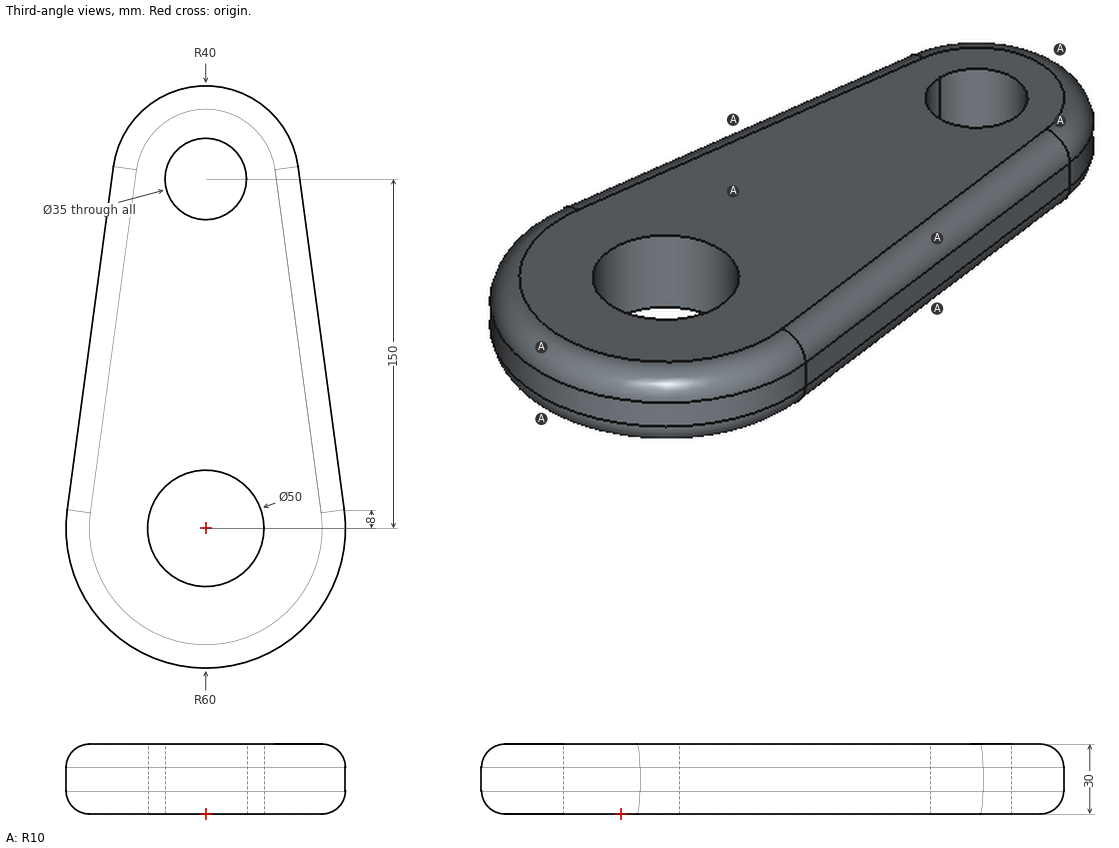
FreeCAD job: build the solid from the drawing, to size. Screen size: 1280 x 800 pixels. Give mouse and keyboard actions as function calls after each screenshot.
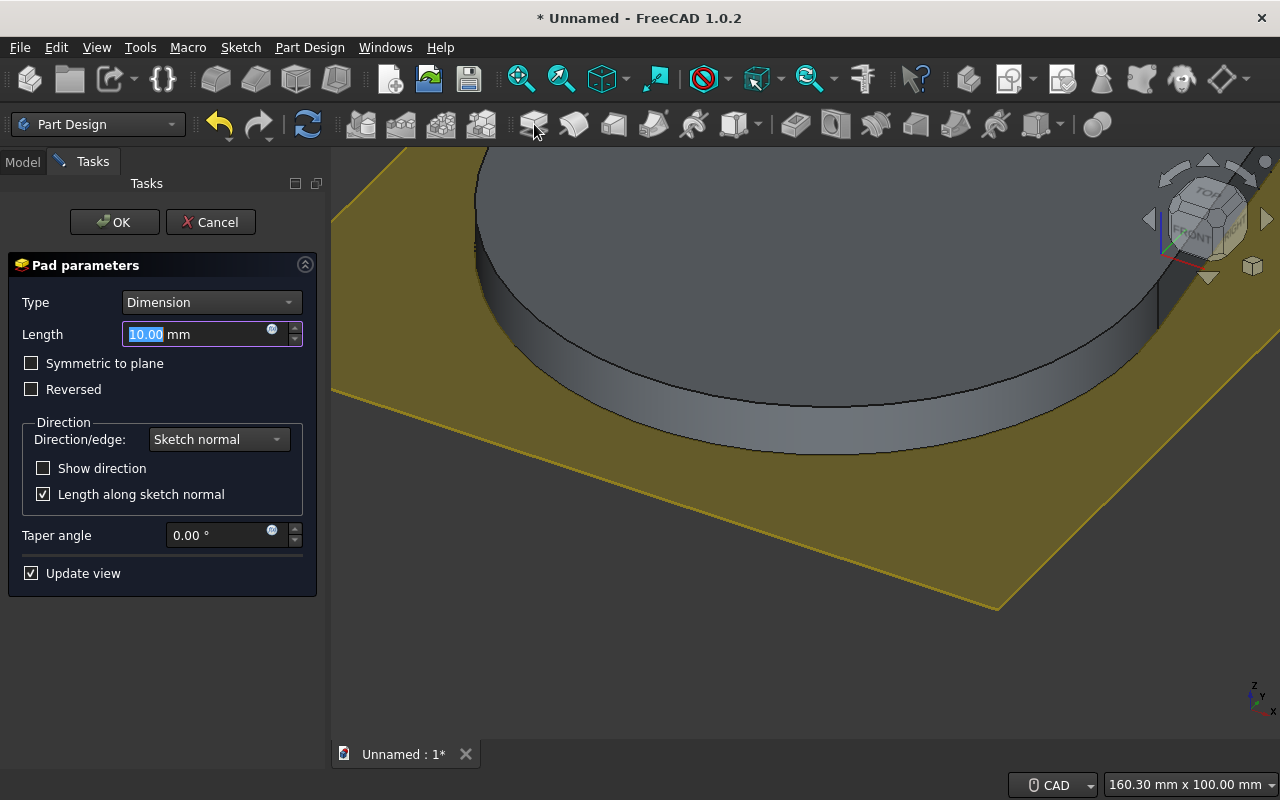
text(30)
key(Tab)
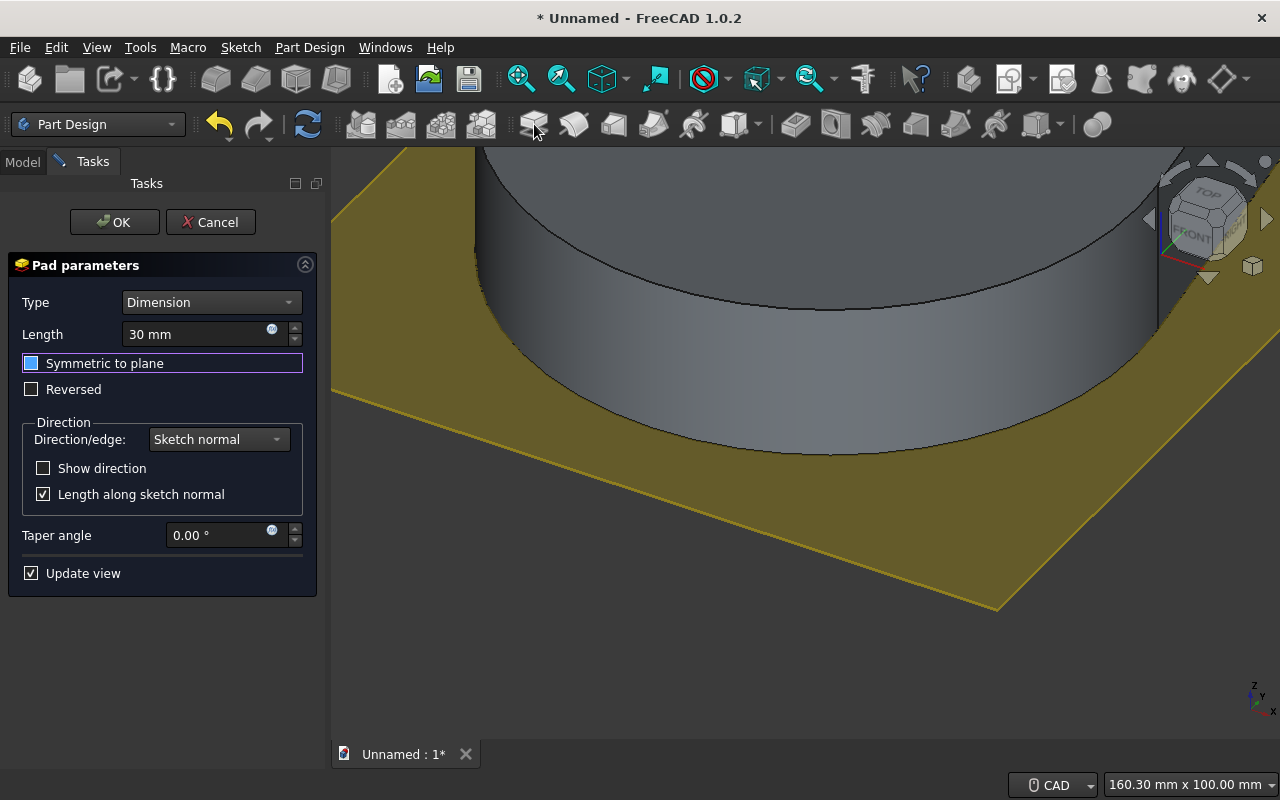
click(30, 389)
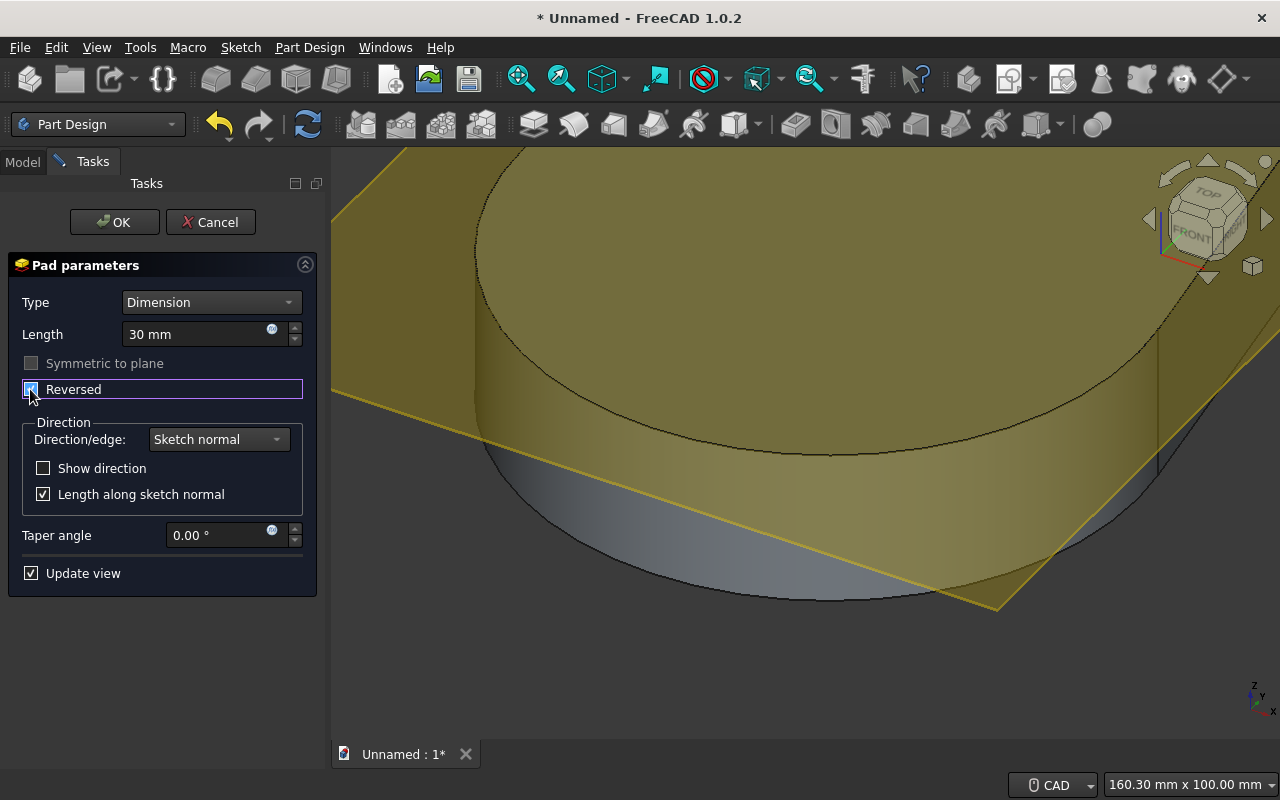
click(115, 222)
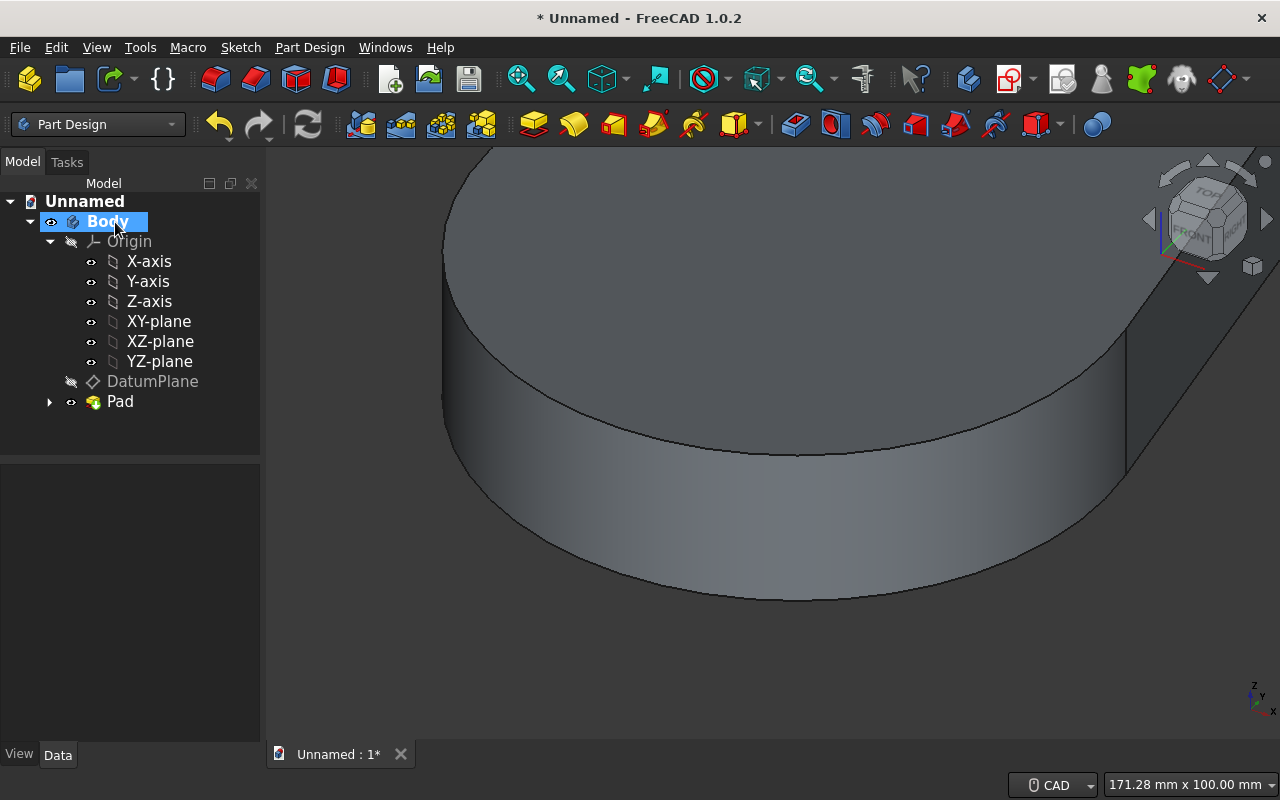
click(522, 80)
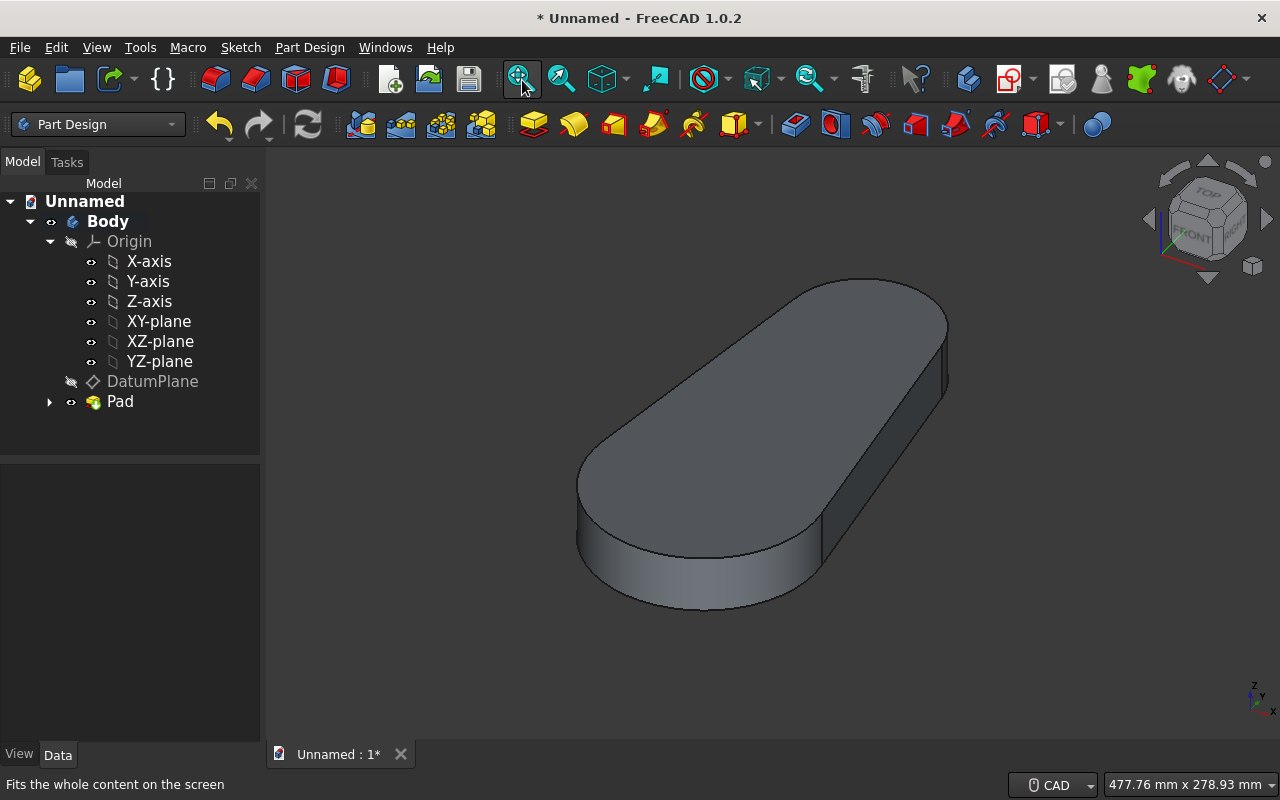
key(5)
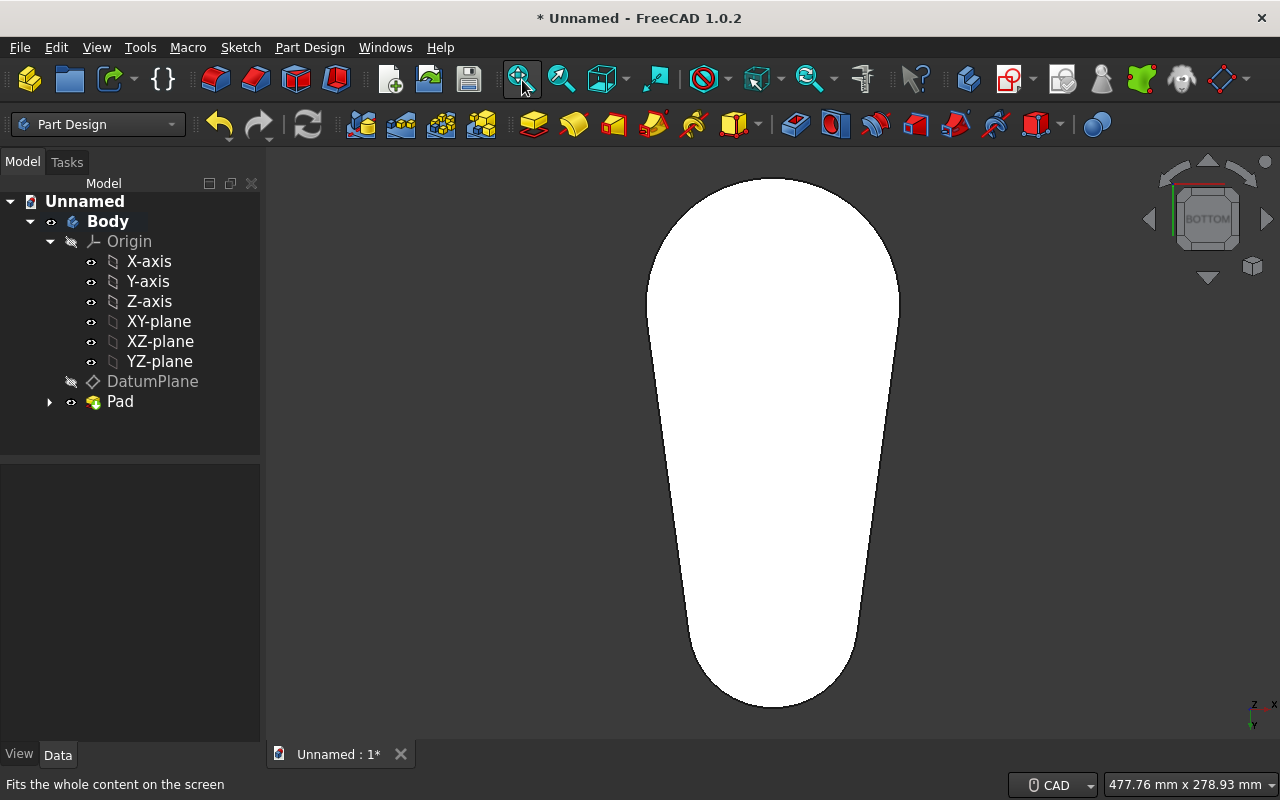
click(773, 366)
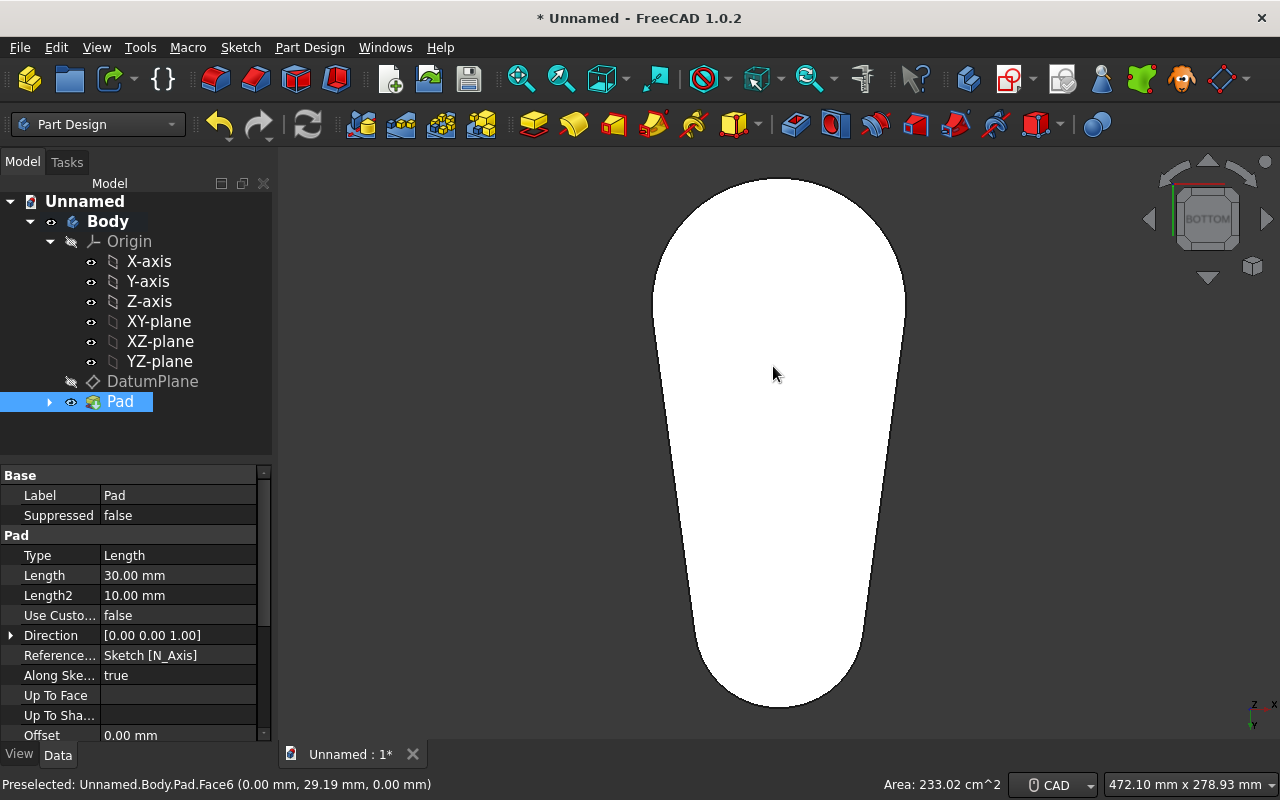
click(1010, 80)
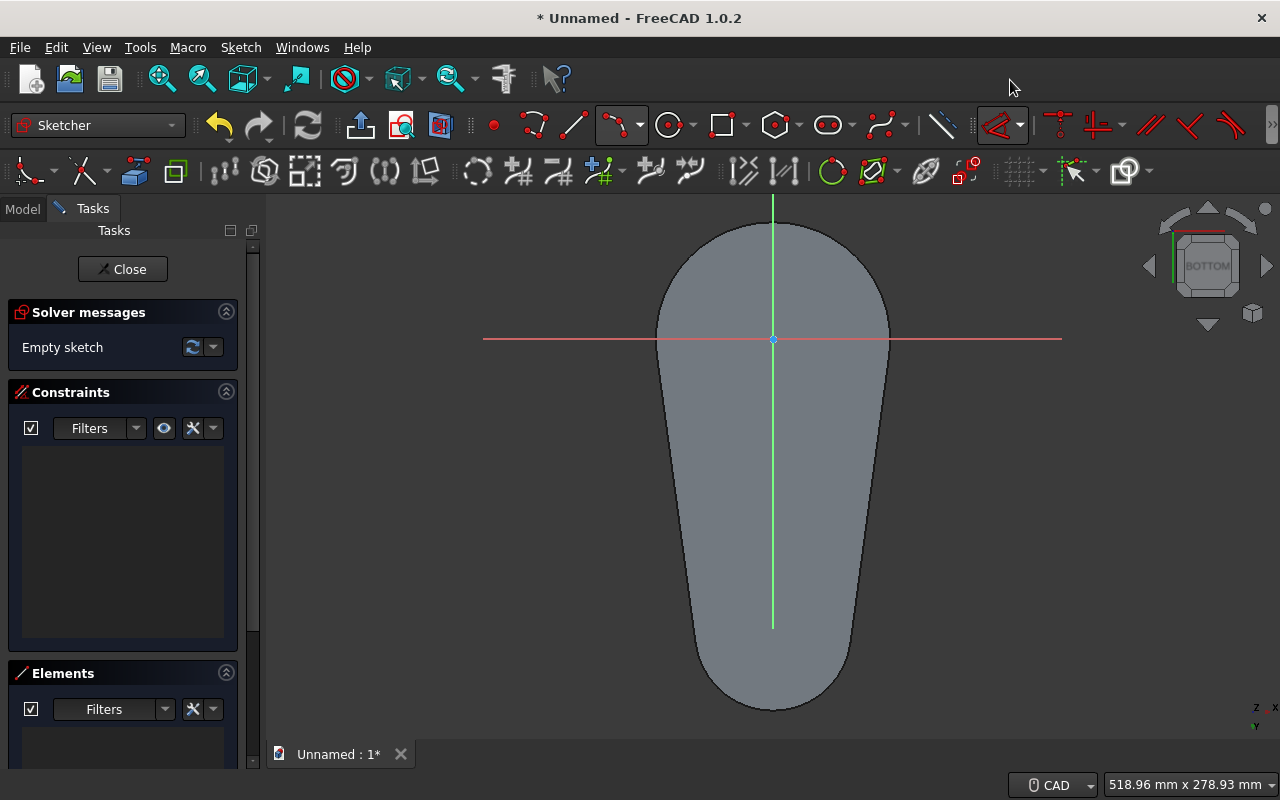
scroll(790, 675, up, 8)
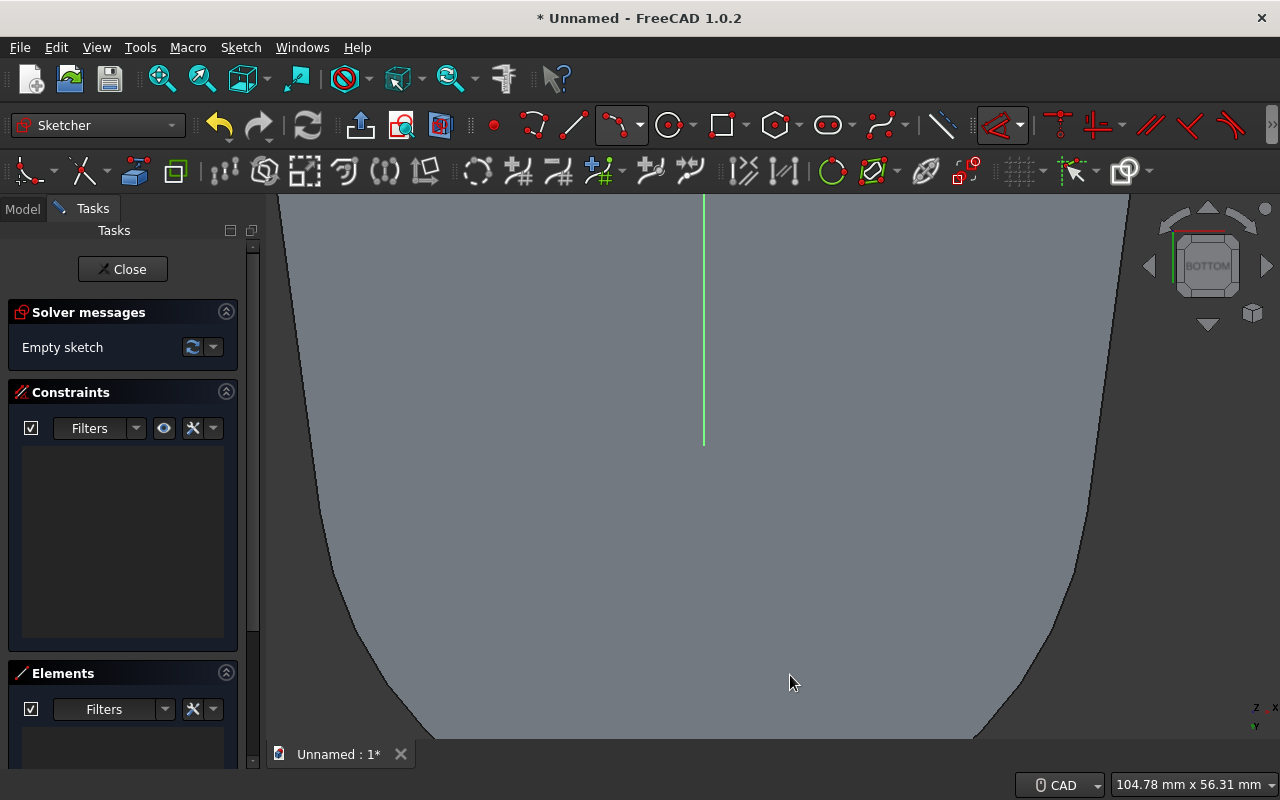
click(670, 126)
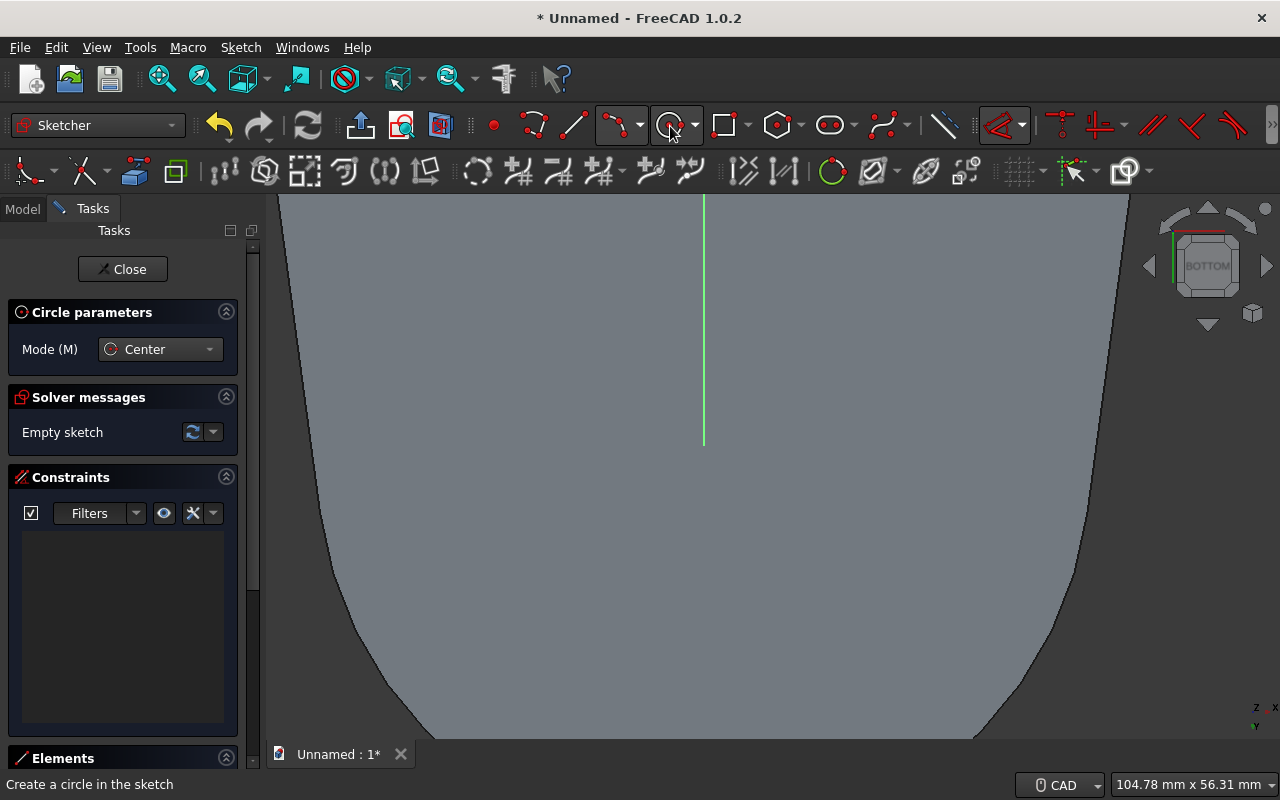
click(704, 461)
click(824, 342)
key(Escape)